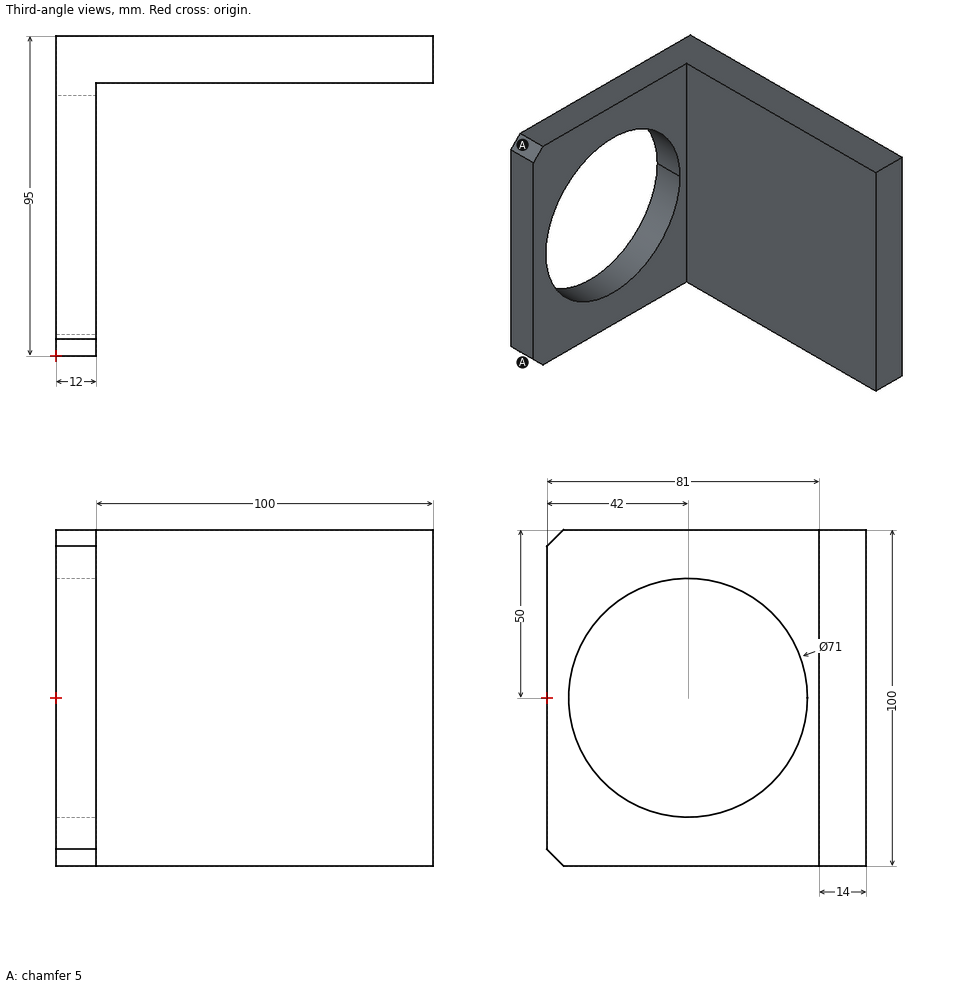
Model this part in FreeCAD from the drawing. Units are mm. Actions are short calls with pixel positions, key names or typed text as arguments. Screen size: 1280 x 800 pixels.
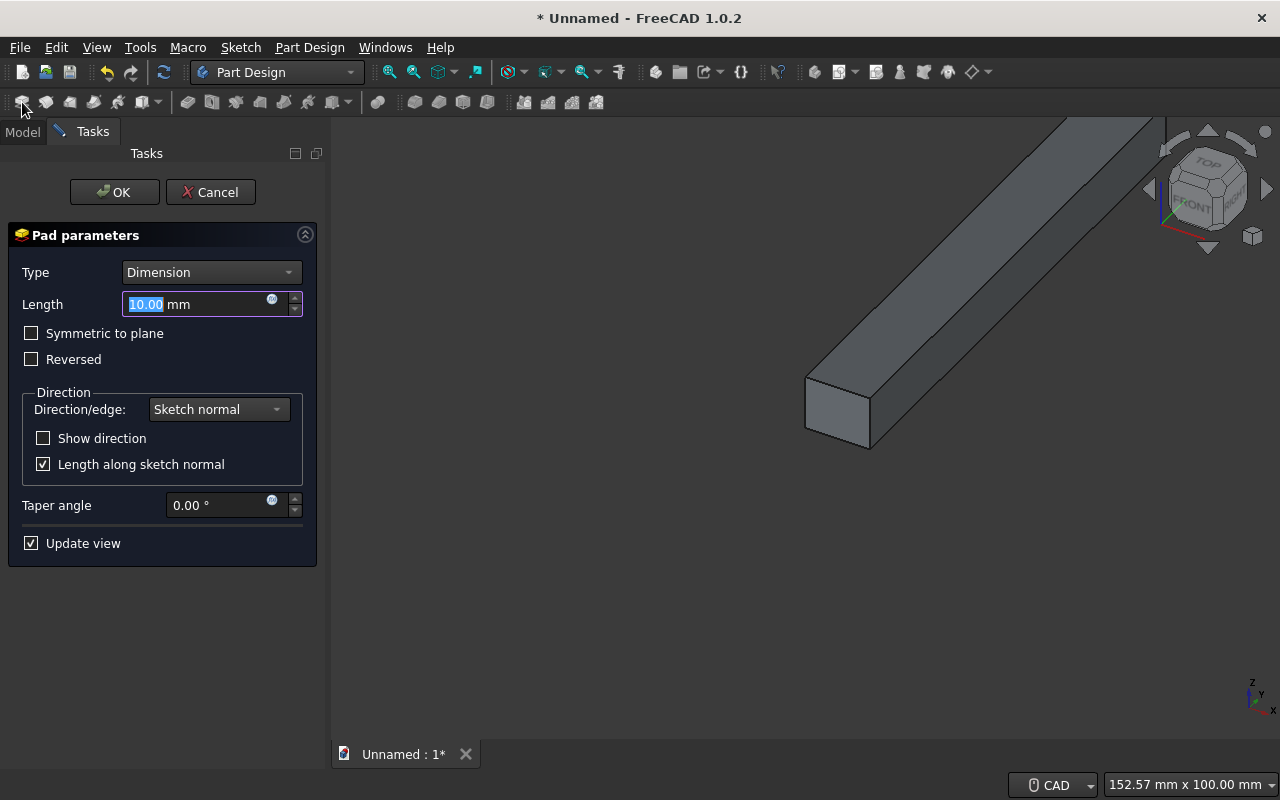
text(100)
key(Tab)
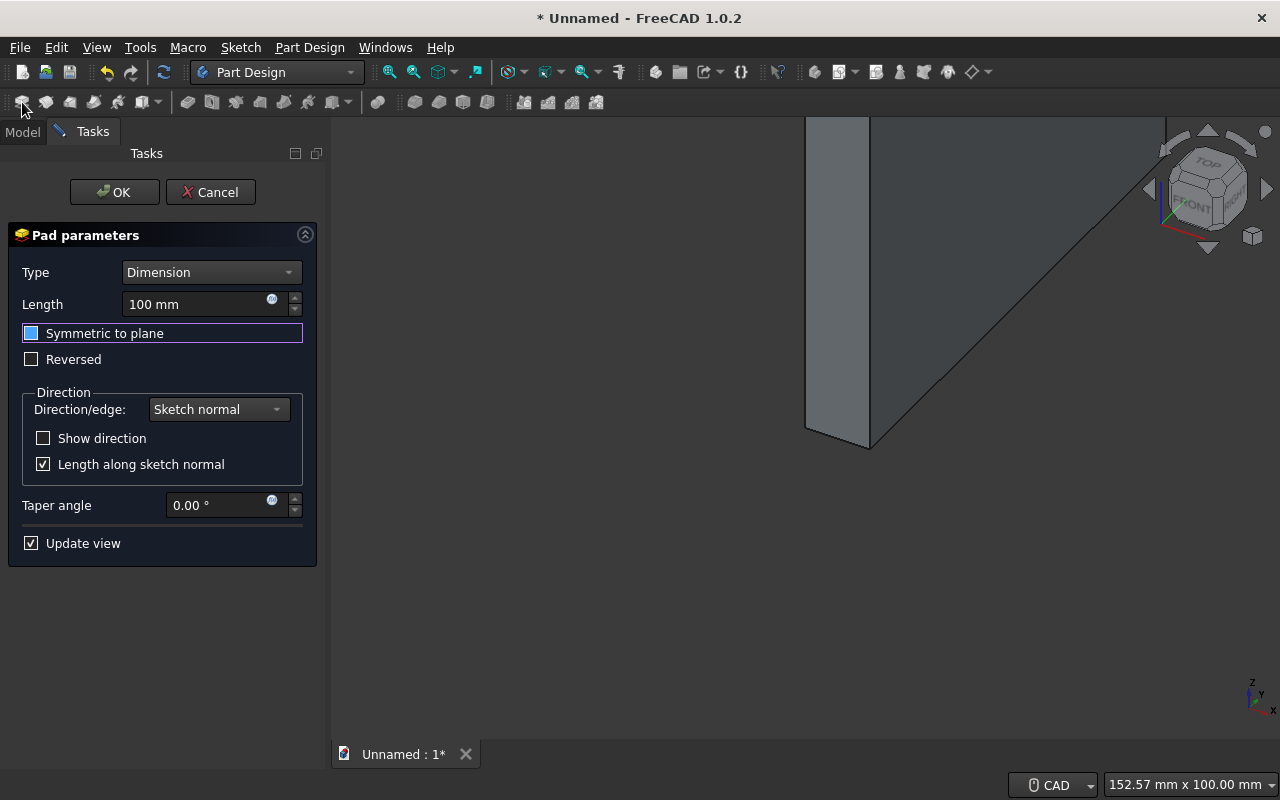
click(30, 333)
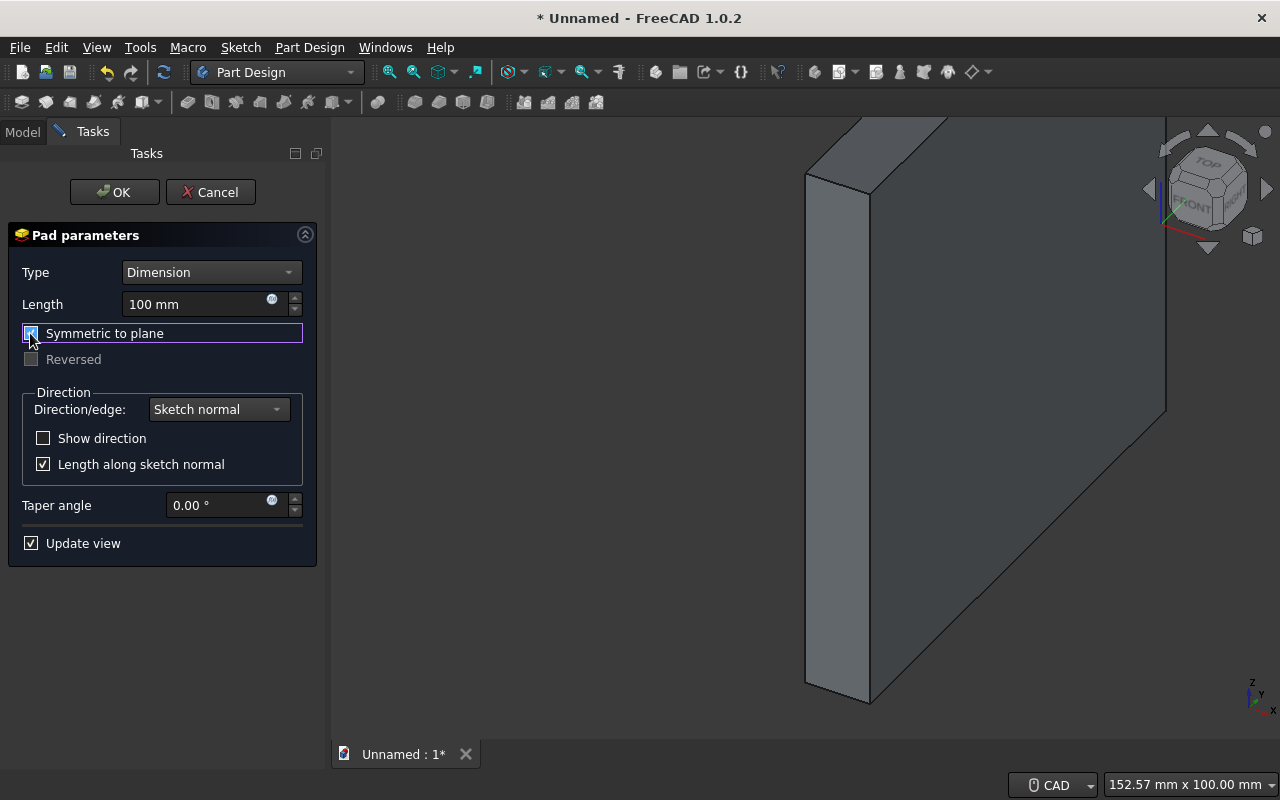
click(115, 192)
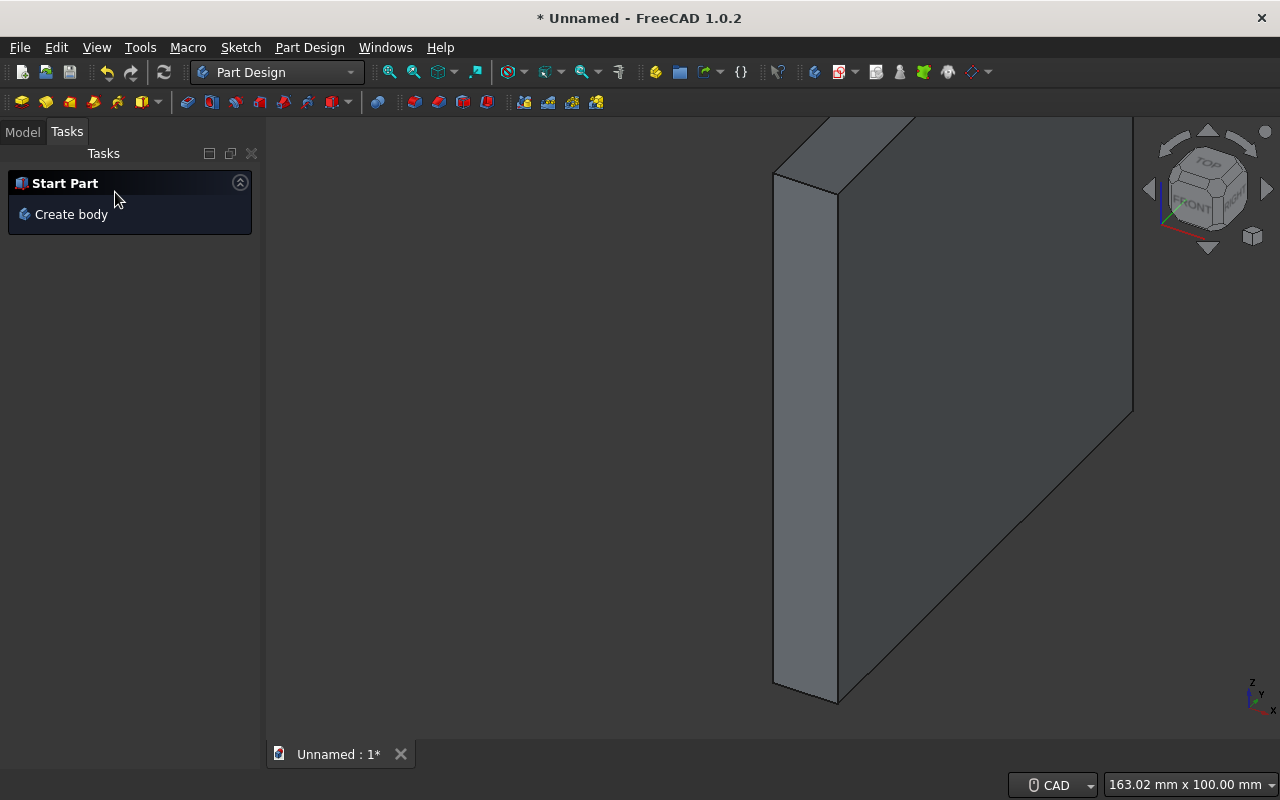
click(390, 72)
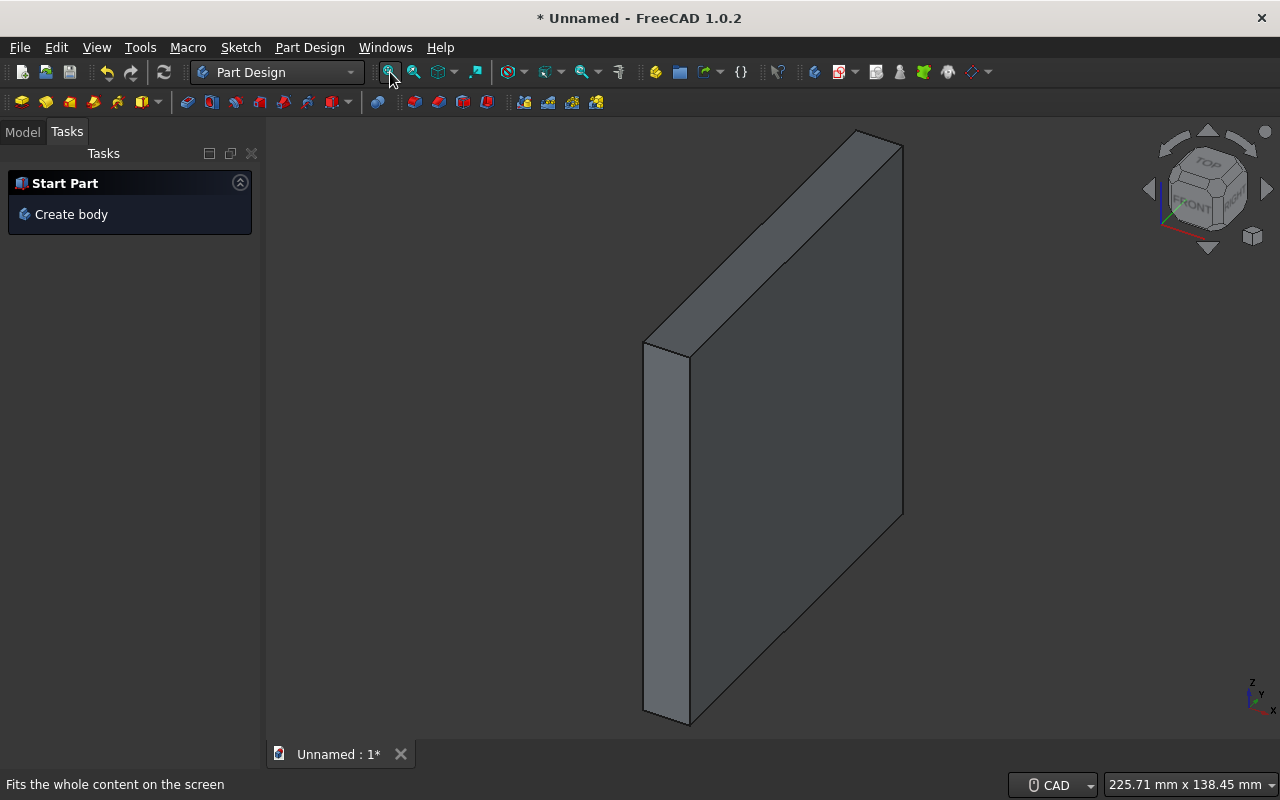
click(796, 435)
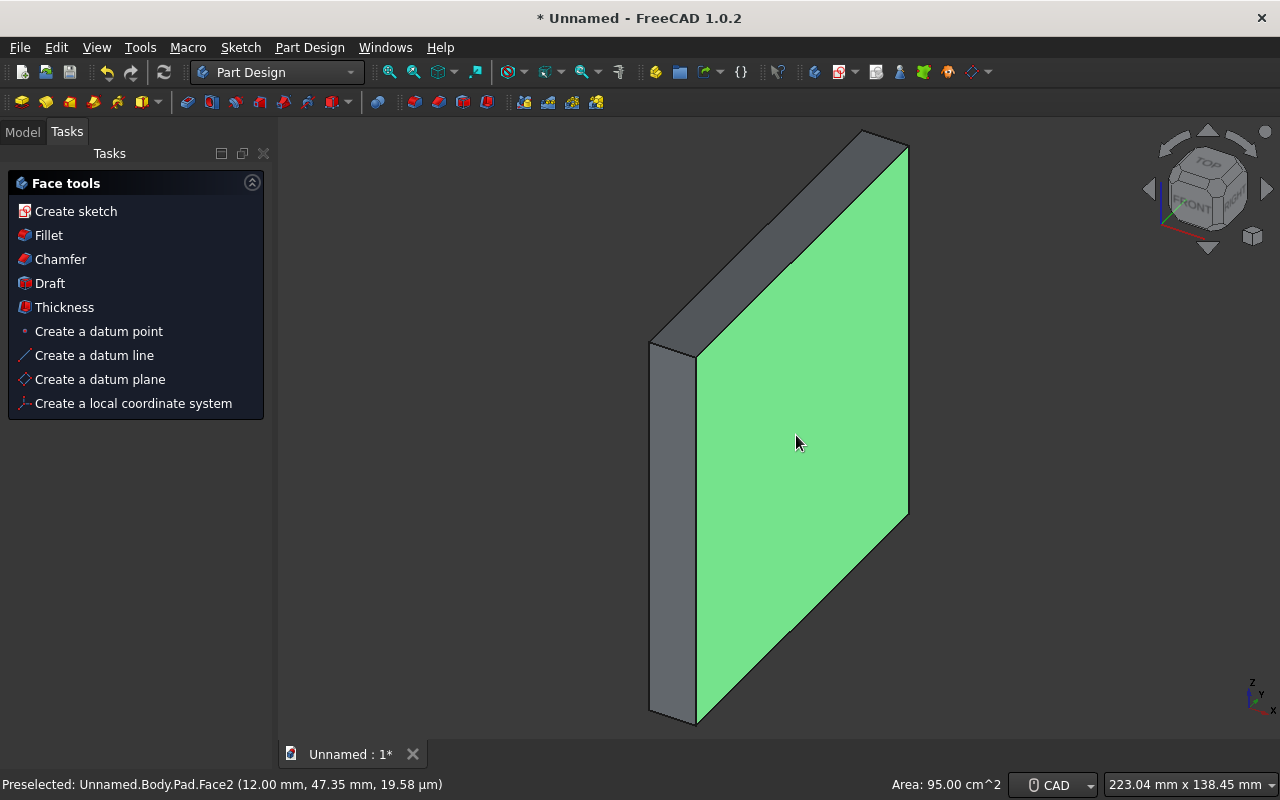
click(840, 72)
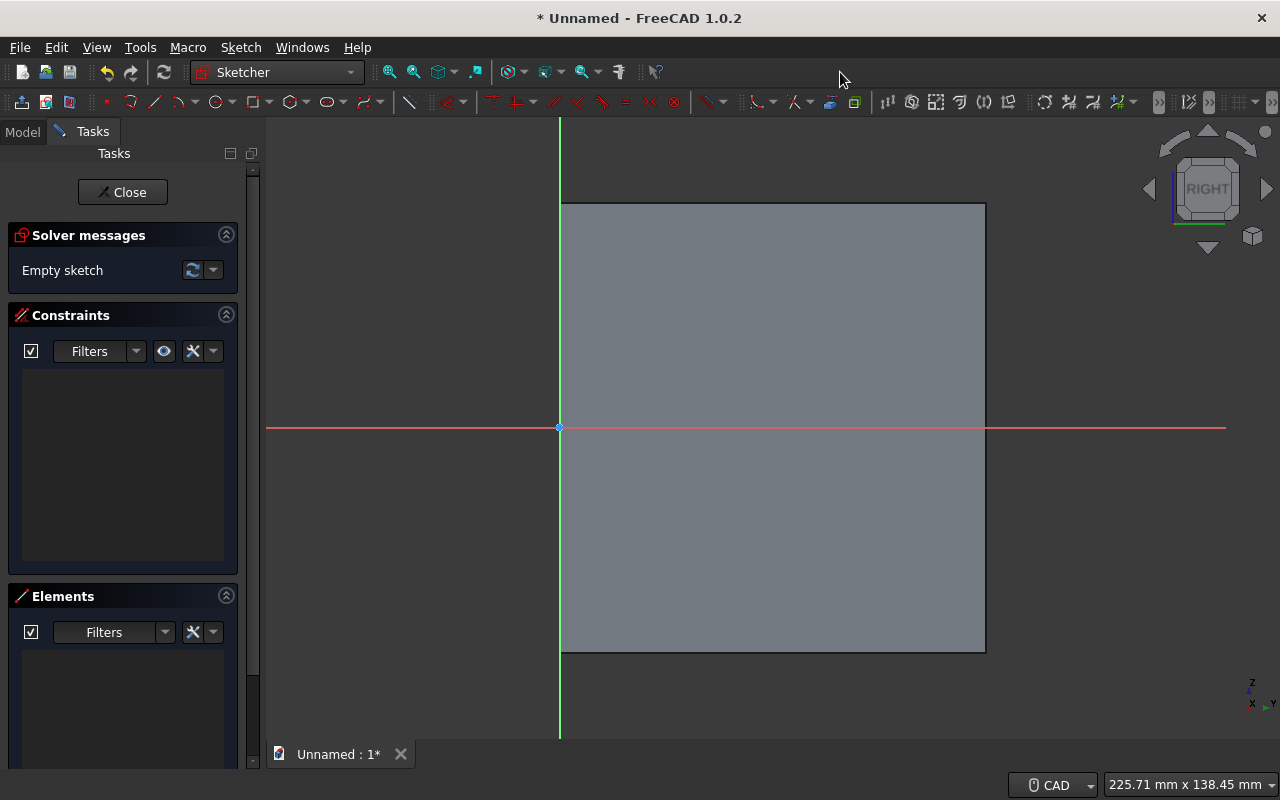
click(216, 102)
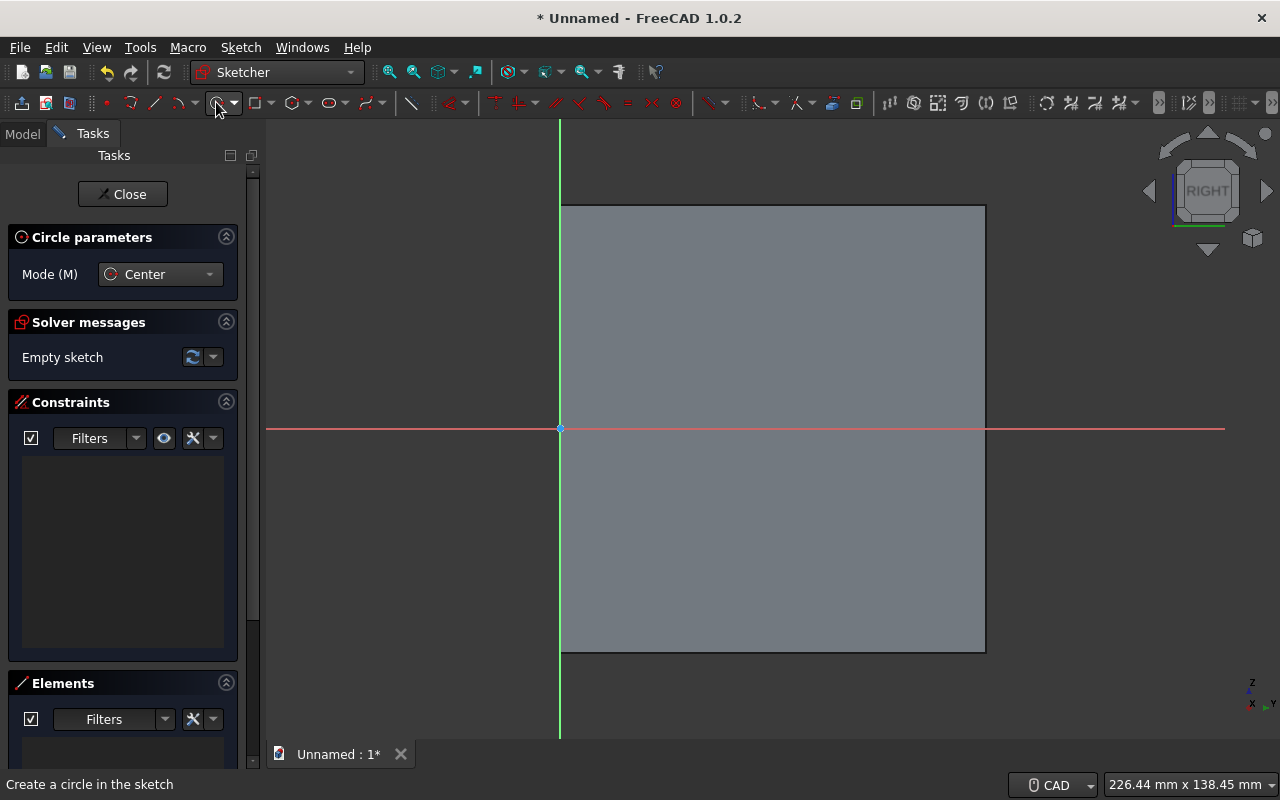
click(748, 429)
move(861, 317)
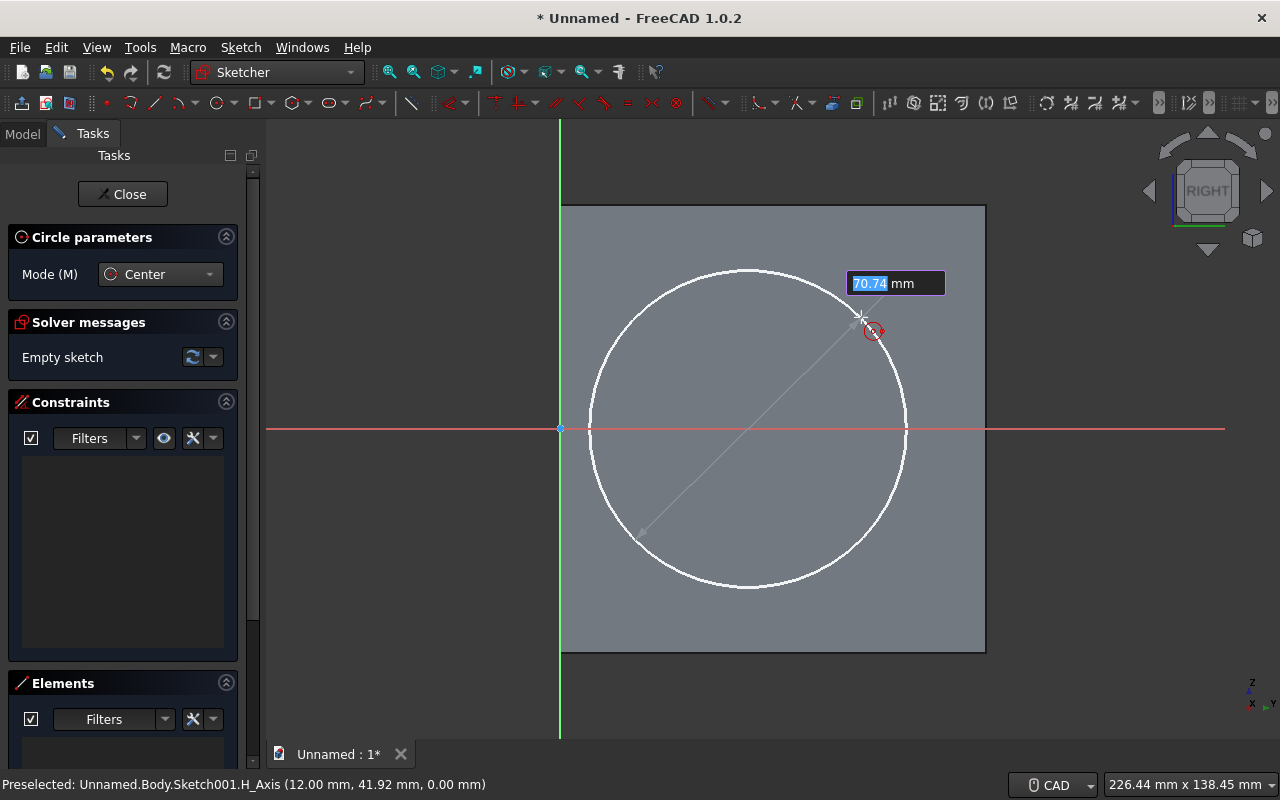
text(71)
key(Return)
key(Escape)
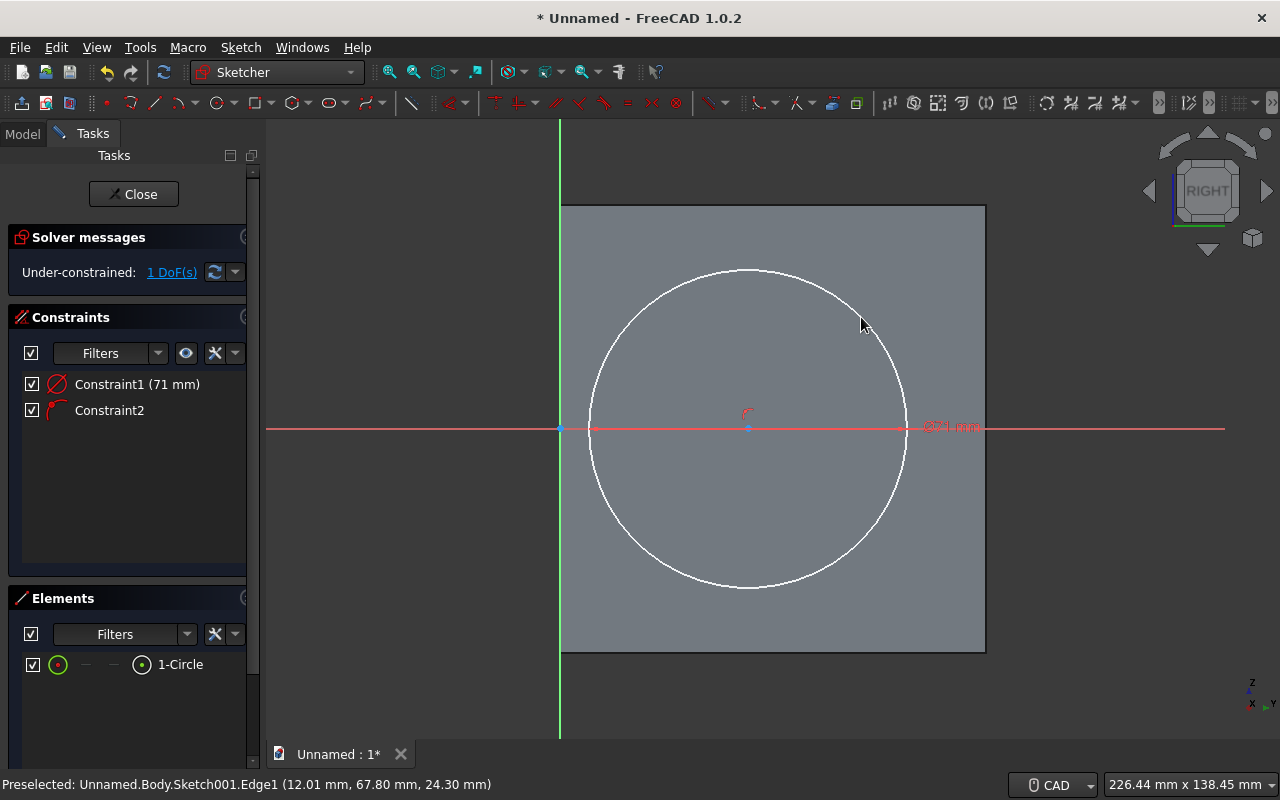
click(450, 104)